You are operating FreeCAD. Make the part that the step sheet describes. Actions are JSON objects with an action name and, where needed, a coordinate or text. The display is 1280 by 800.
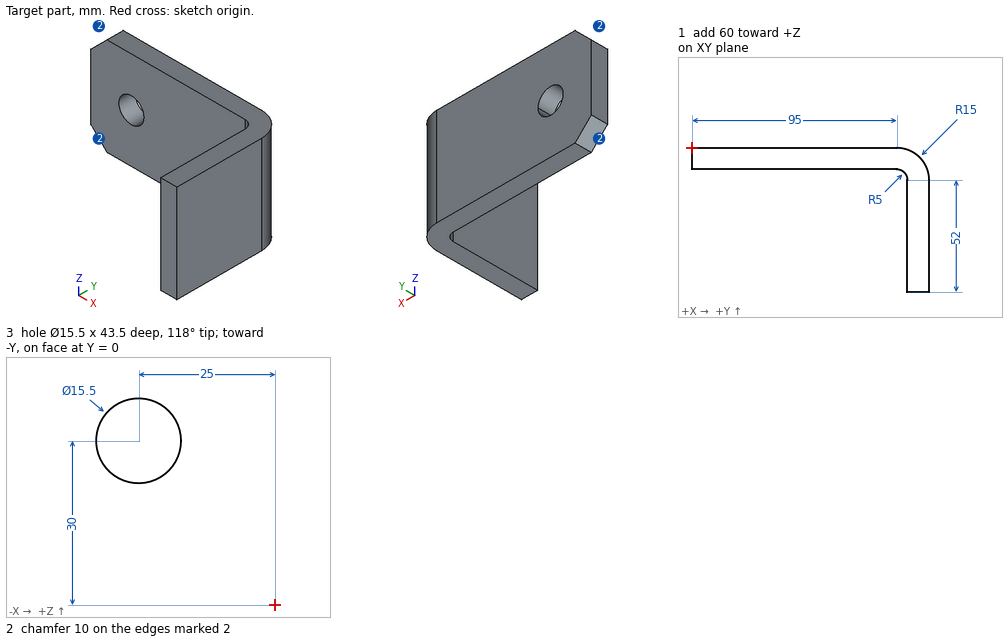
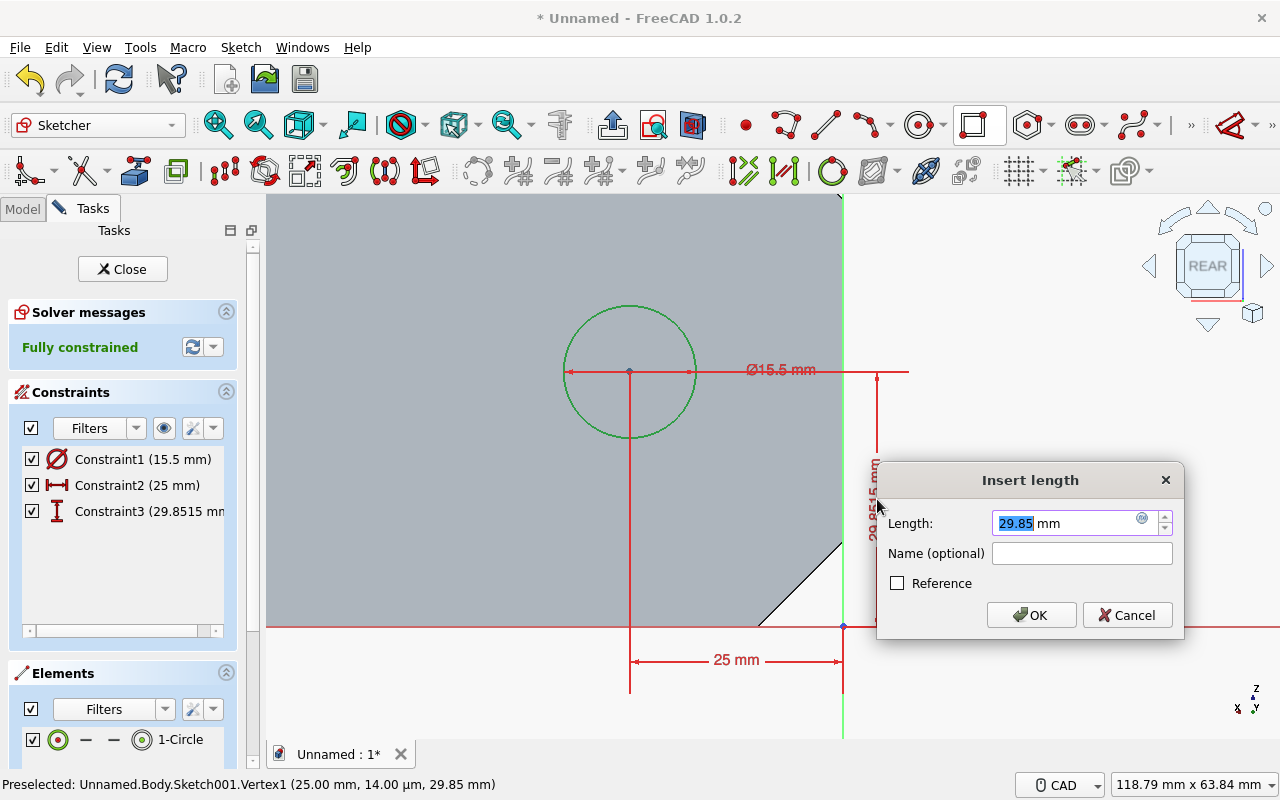
{"action": "type", "text": "30"}
{"action": "key", "text": "Return"}
{"action": "key", "text": "Escape"}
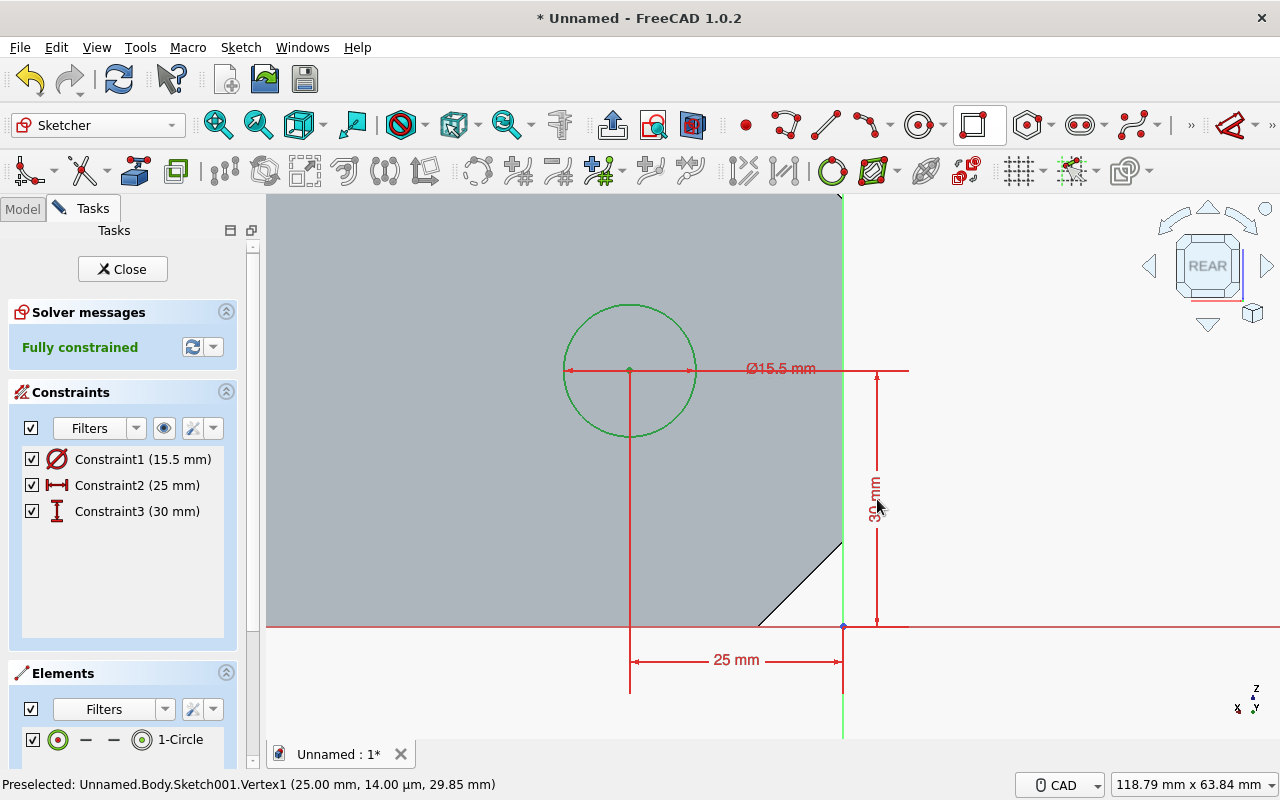
{"action": "left_click", "coordinate": [123, 269]}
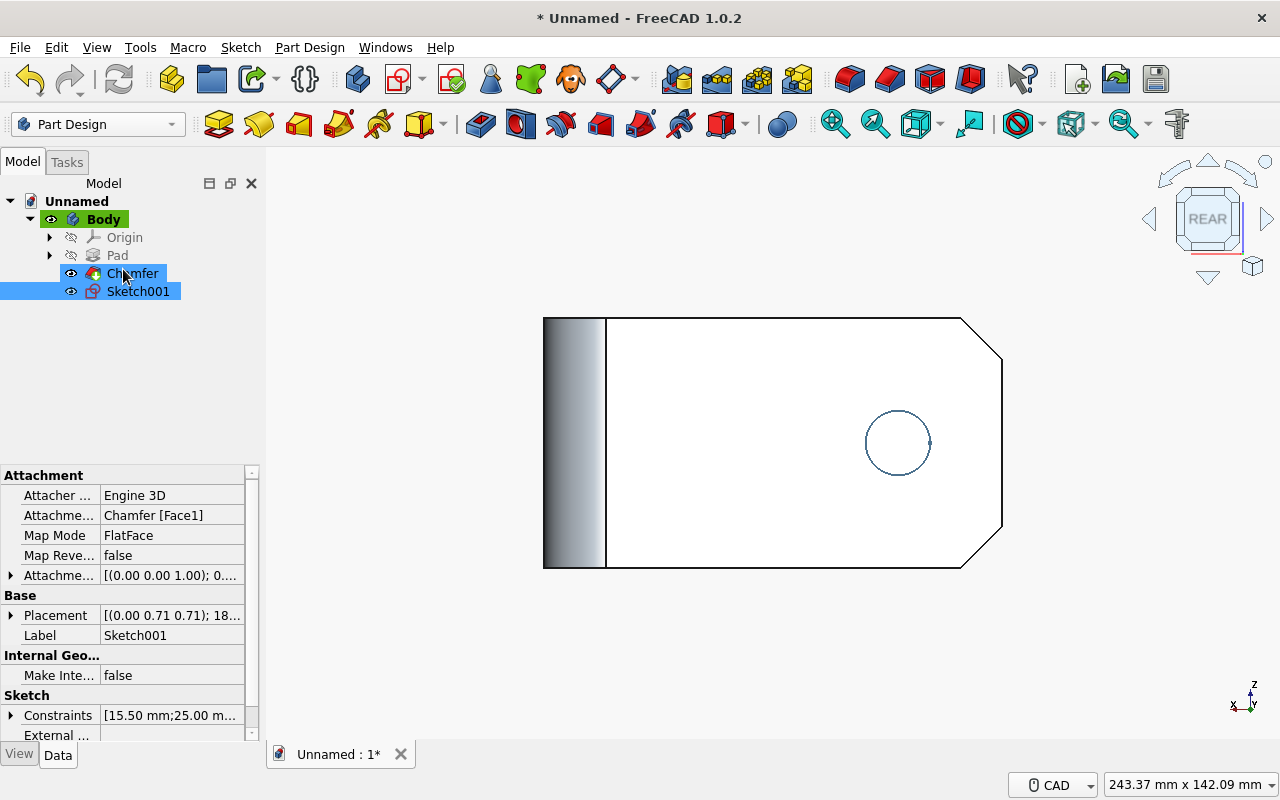
{"action": "left_click", "coordinate": [522, 124]}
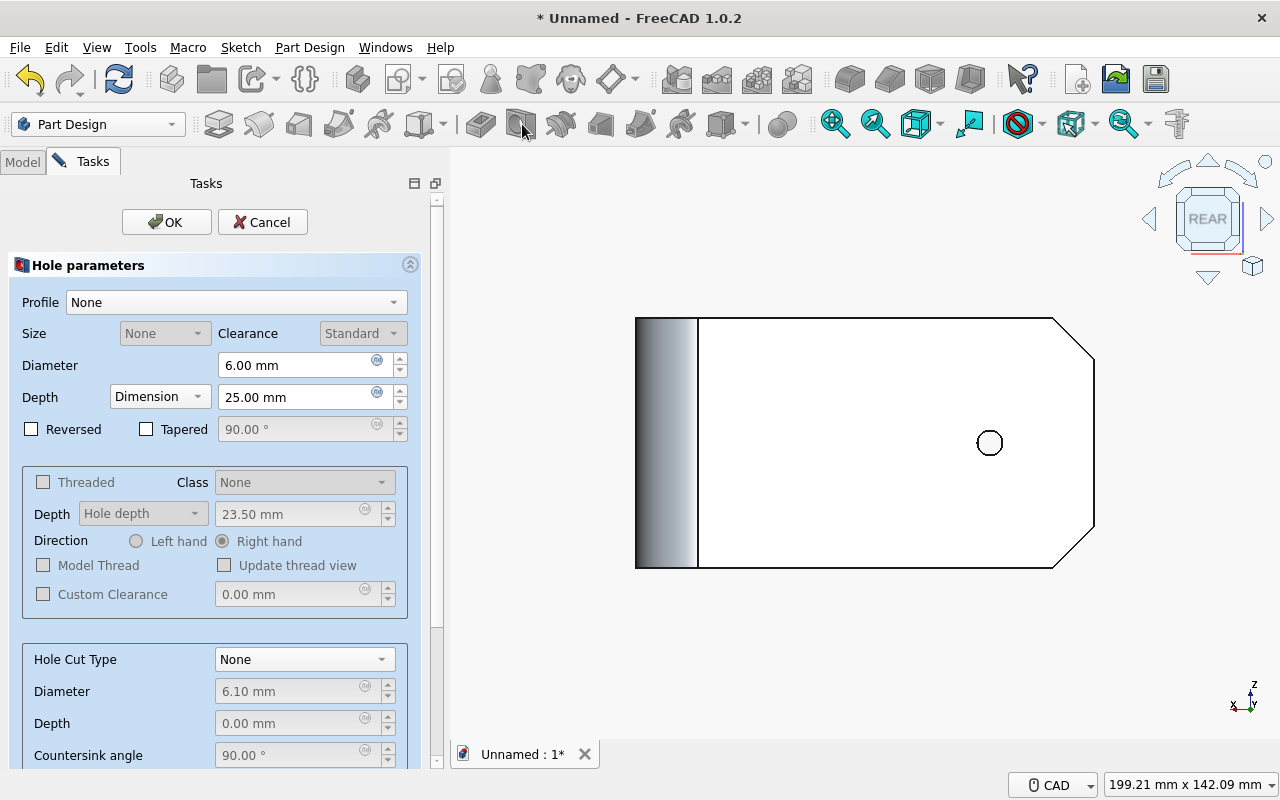
{"action": "triple_click", "coordinate": [305, 365]}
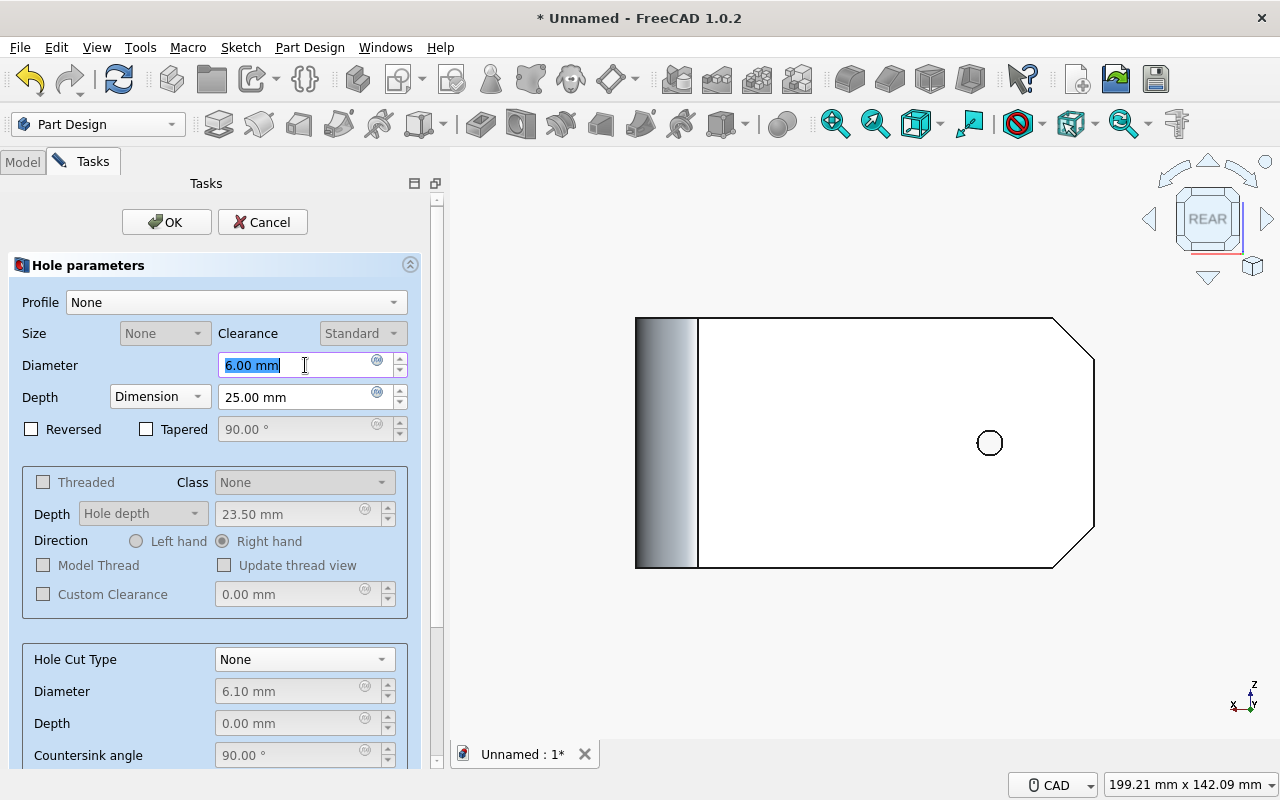
{"action": "type", "text": "15.5"}
{"action": "key", "text": "Tab"}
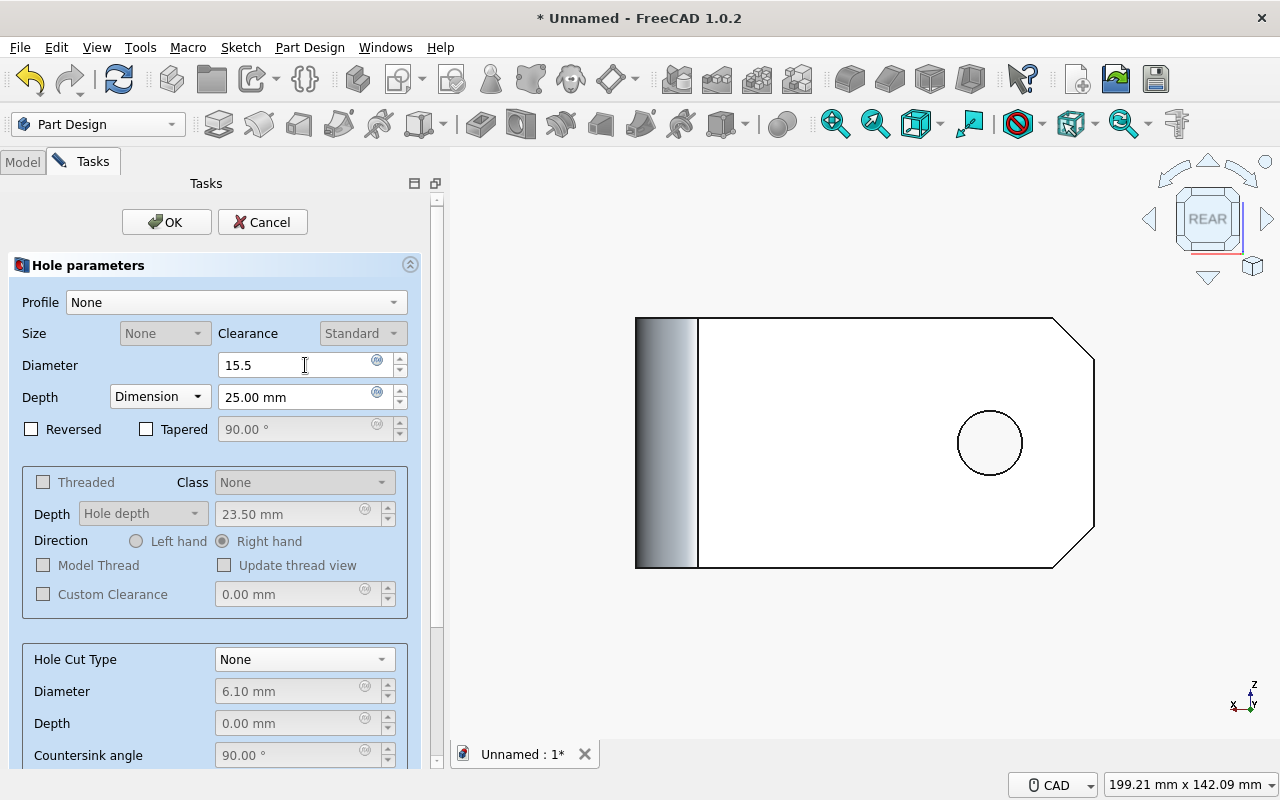
{"action": "triple_click", "coordinate": [305, 397]}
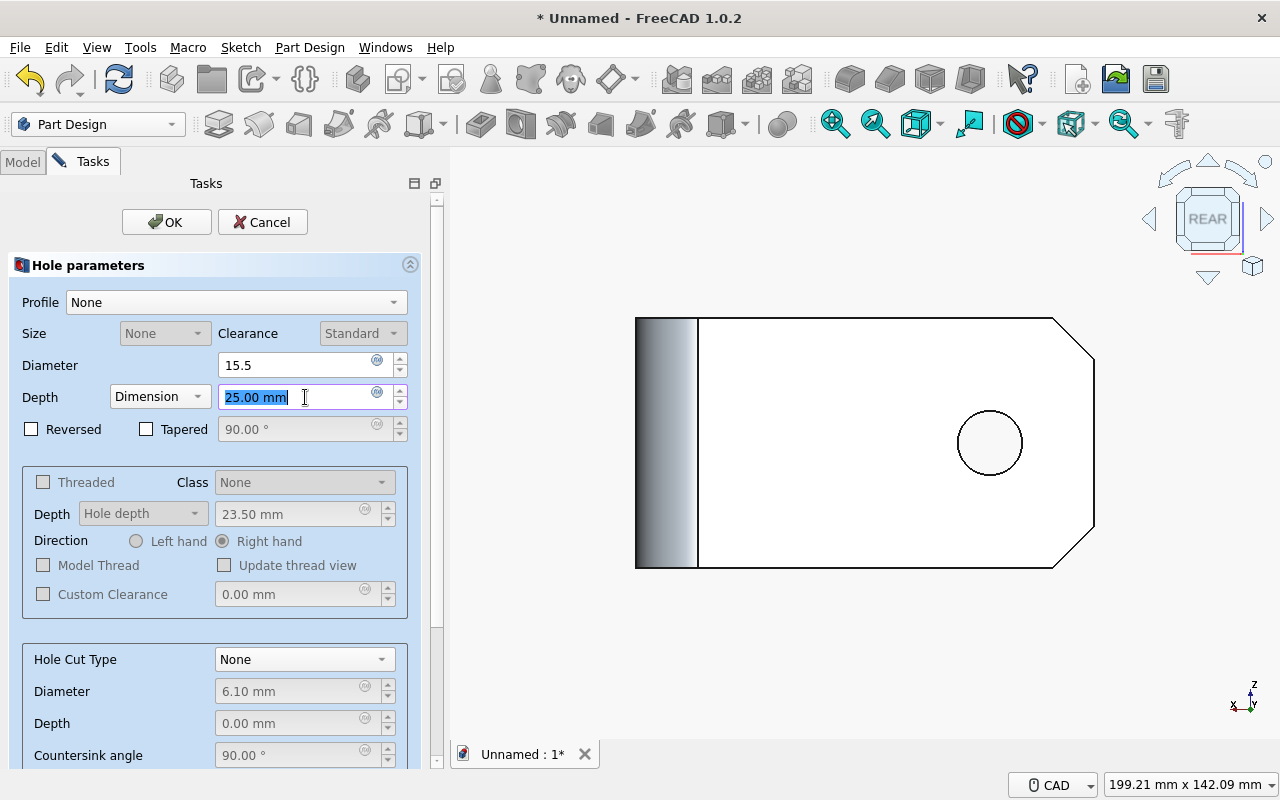
{"action": "type", "text": "43.5"}
{"action": "key", "text": "Tab"}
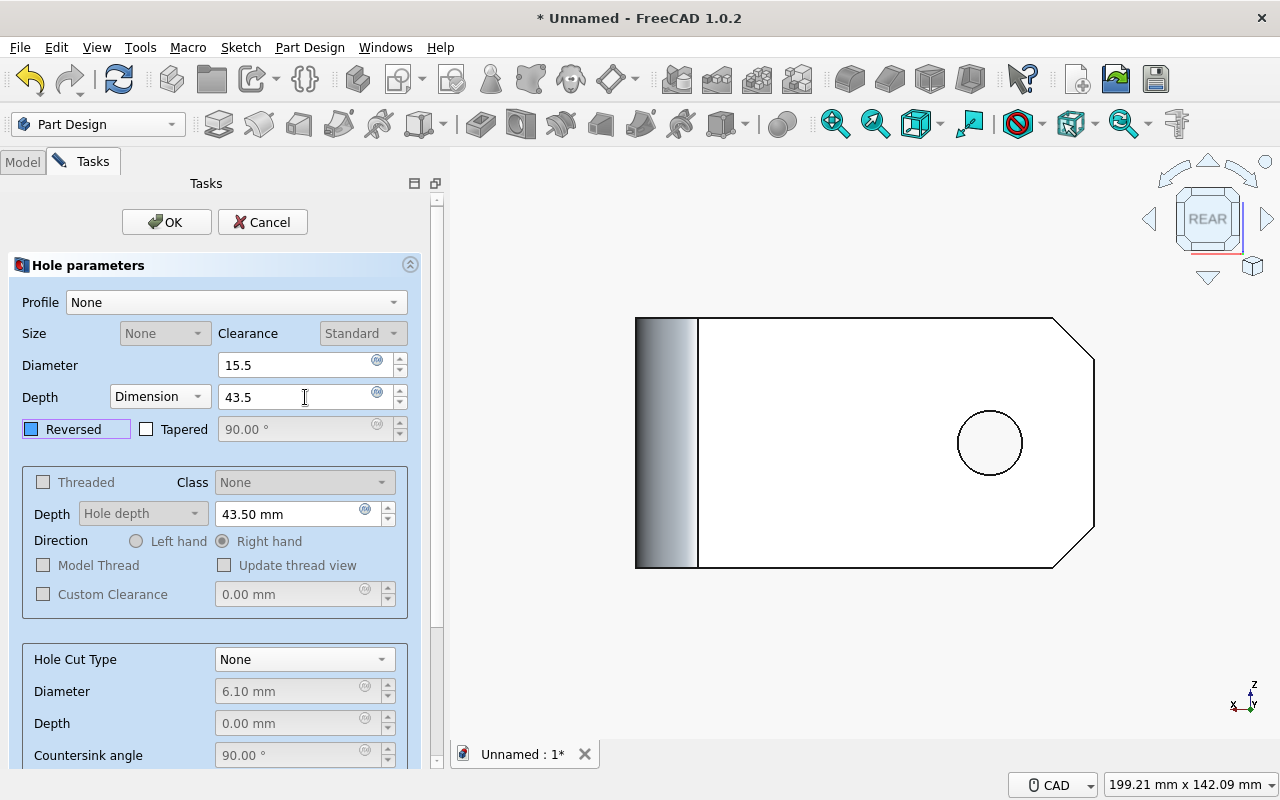
{"action": "left_click", "coordinate": [167, 222]}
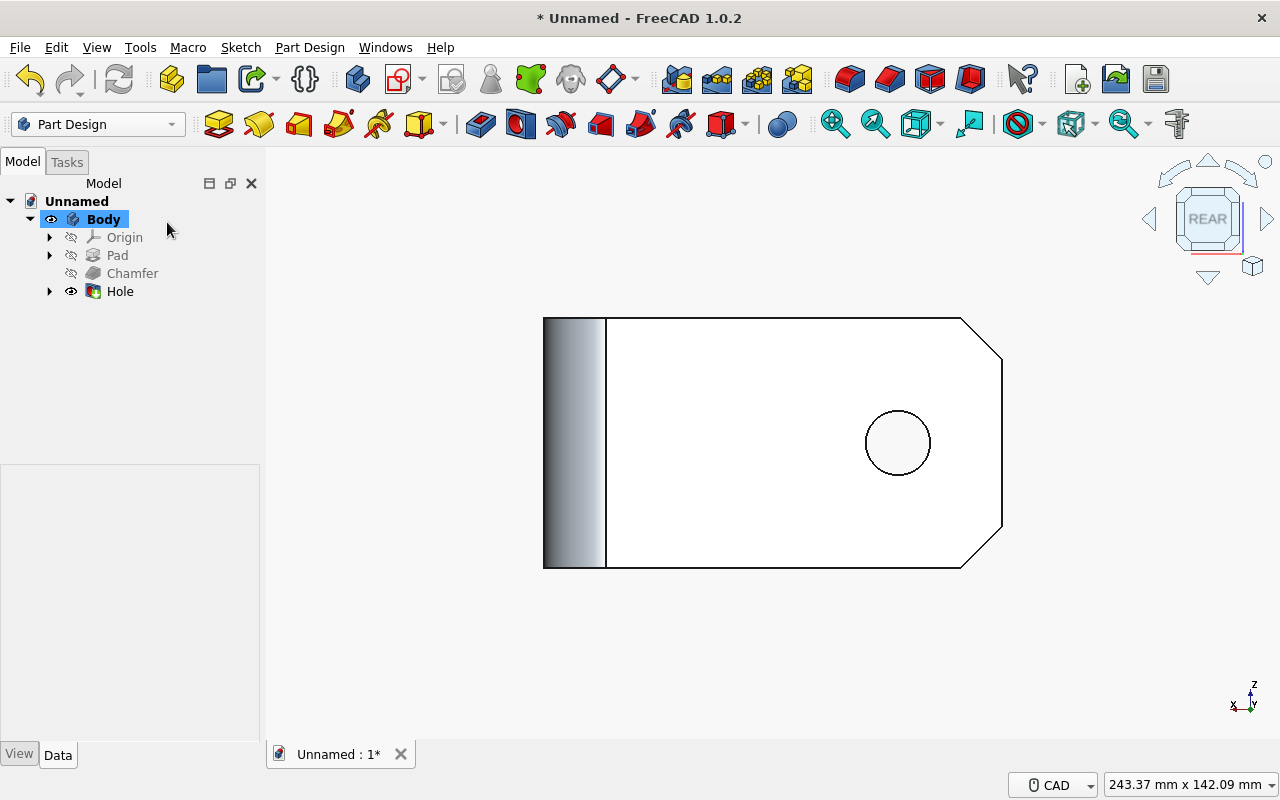
{"action": "key", "text": "0"}